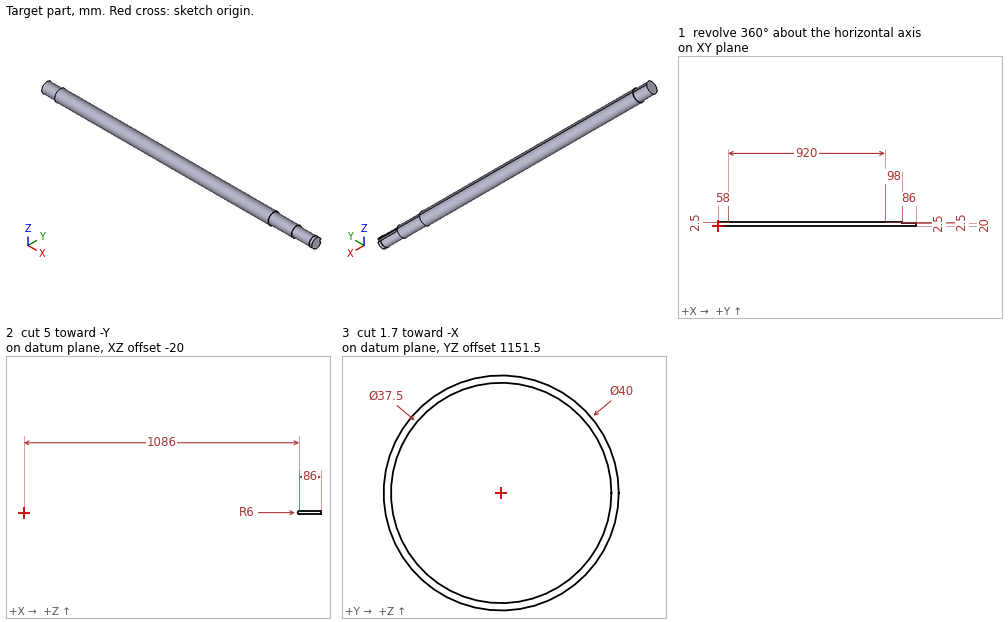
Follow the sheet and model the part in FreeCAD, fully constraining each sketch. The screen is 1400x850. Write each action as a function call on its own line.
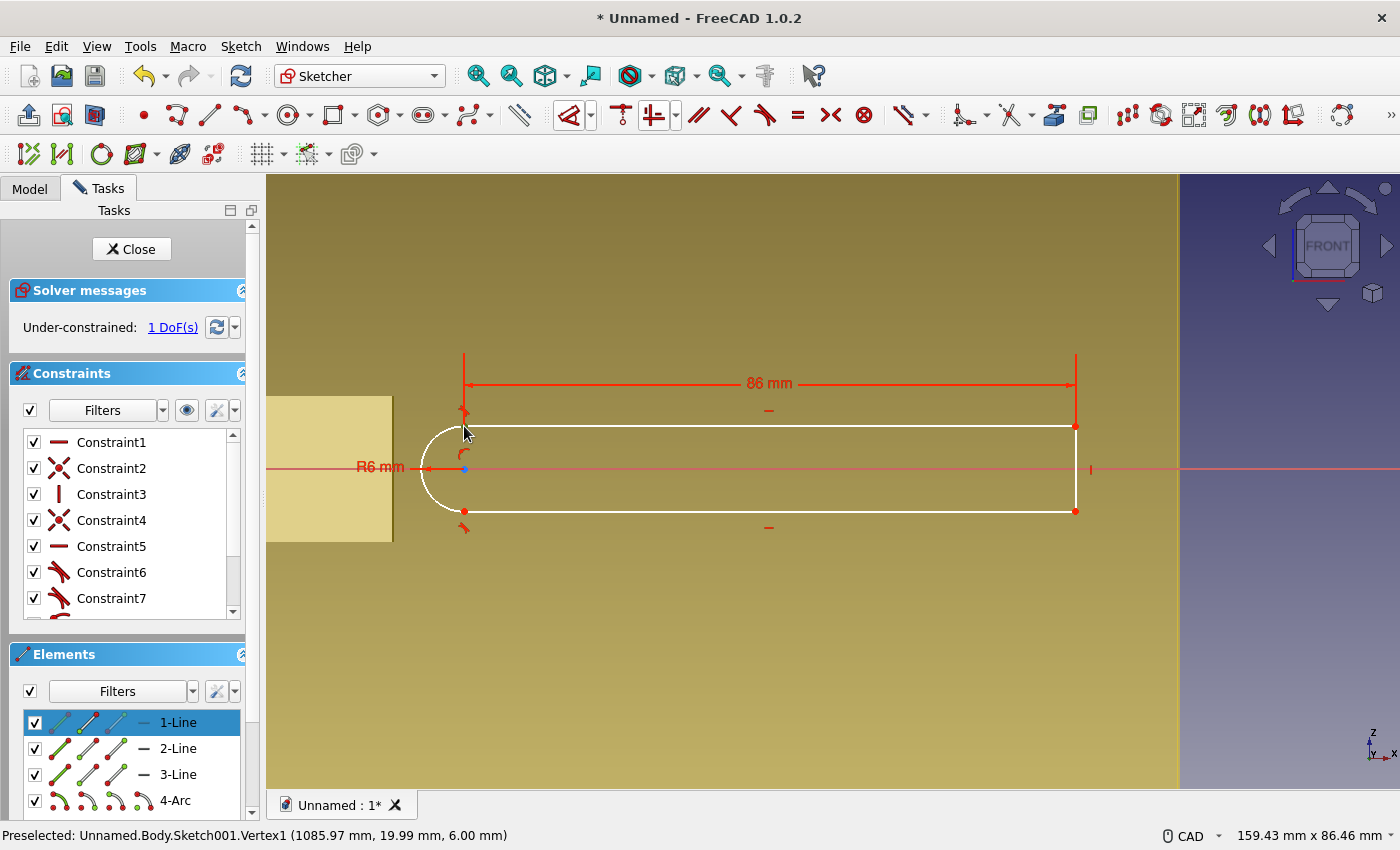
click(590, 116)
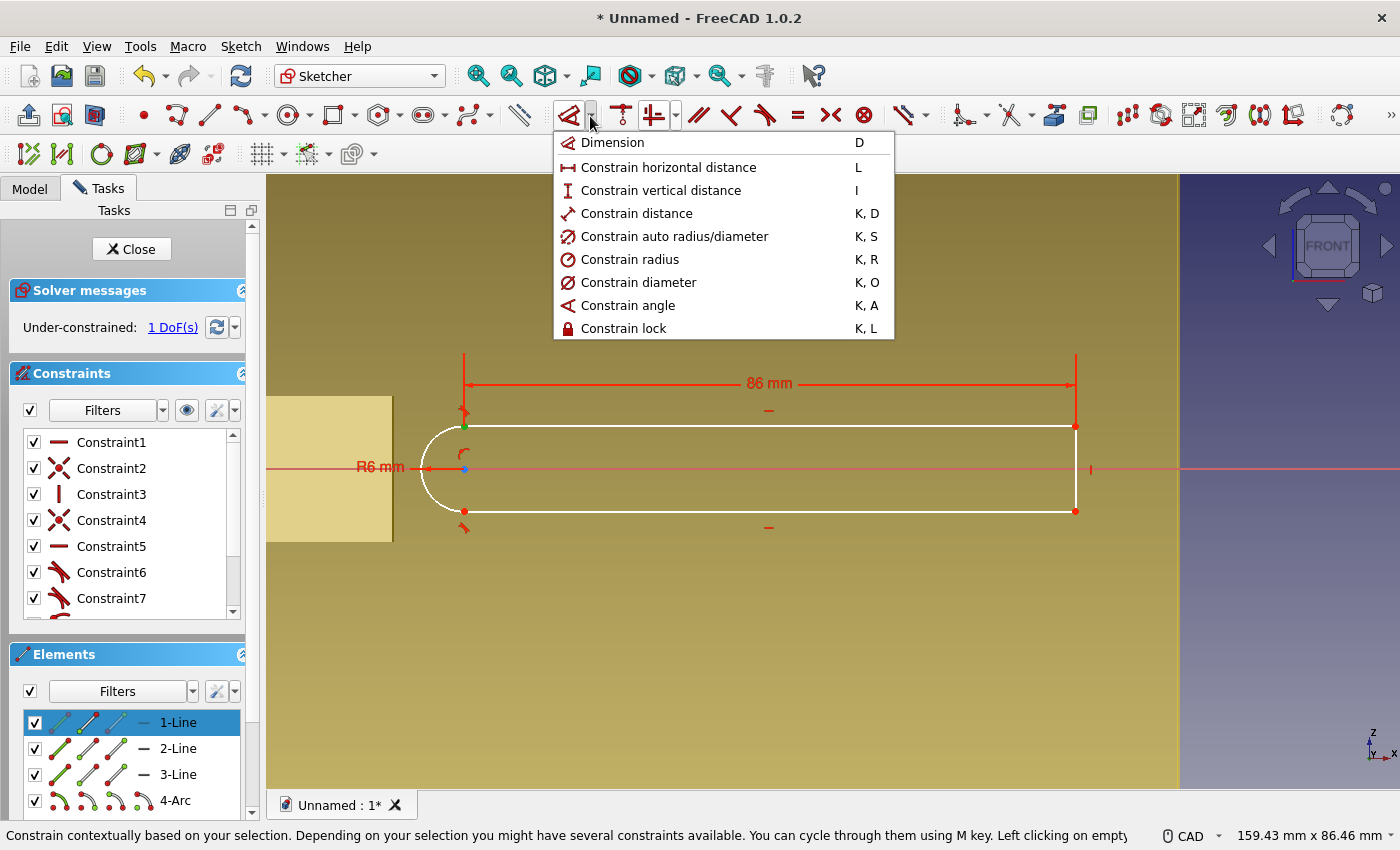
click(724, 168)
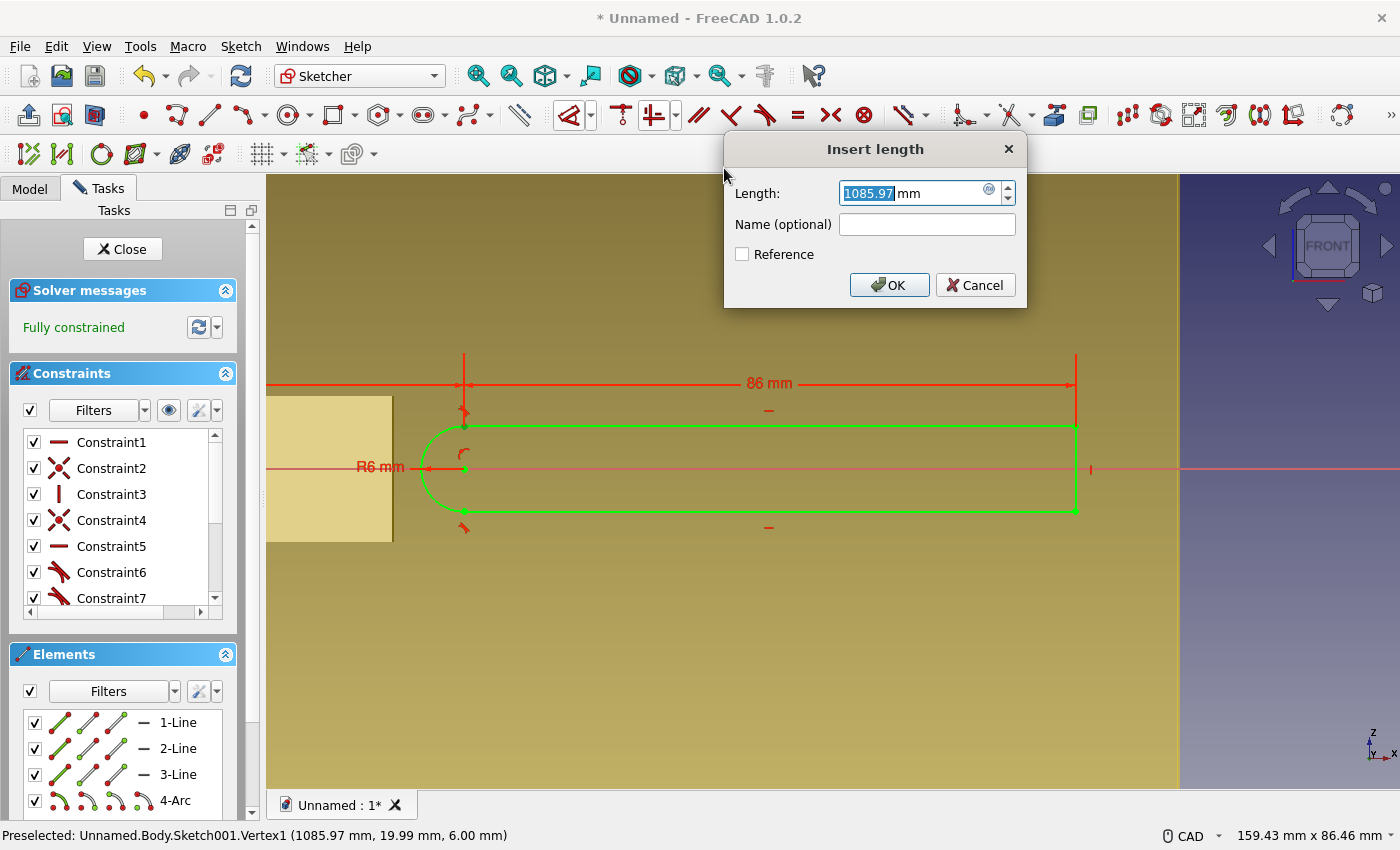
text(1086)
key(Return)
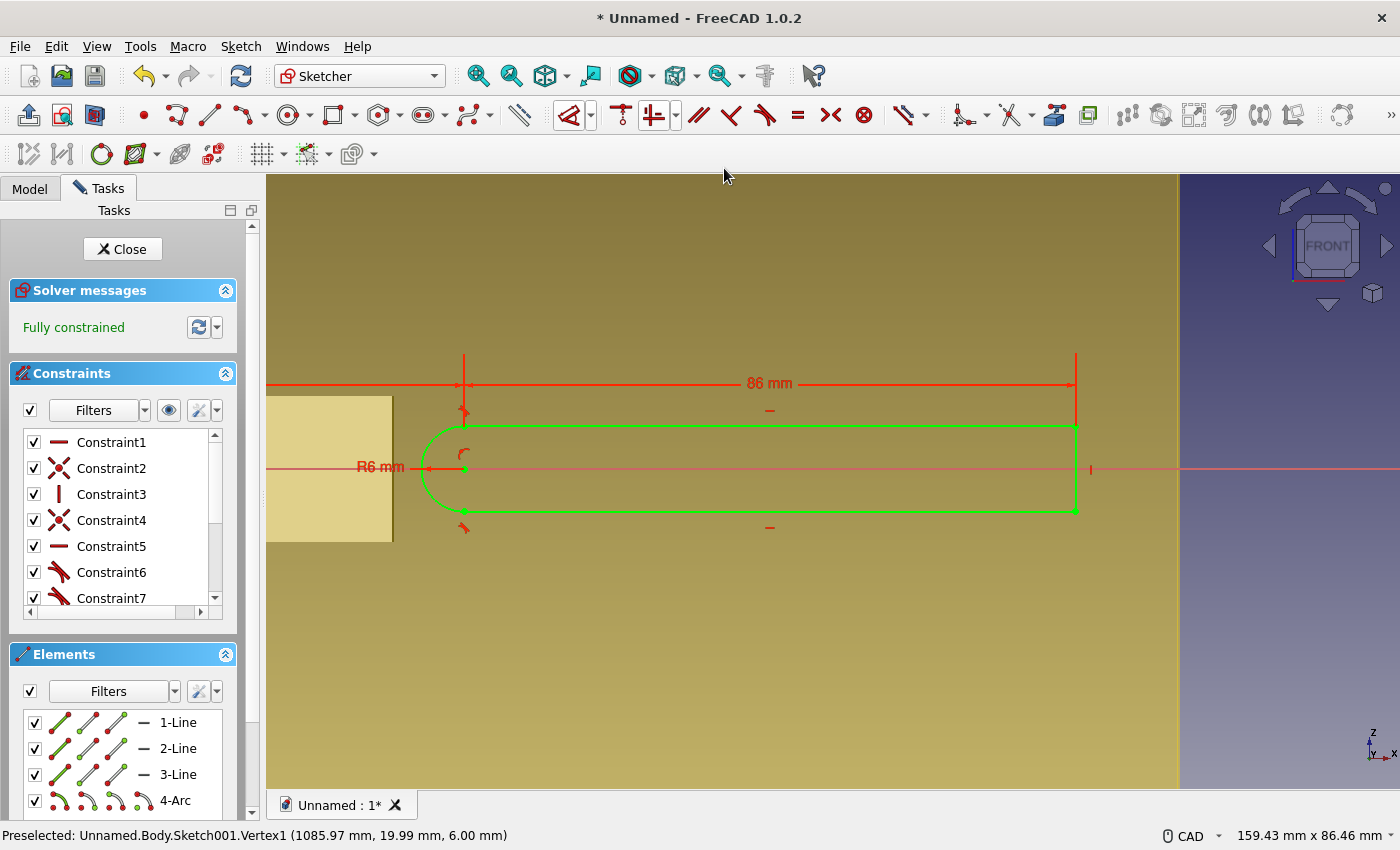
click(123, 249)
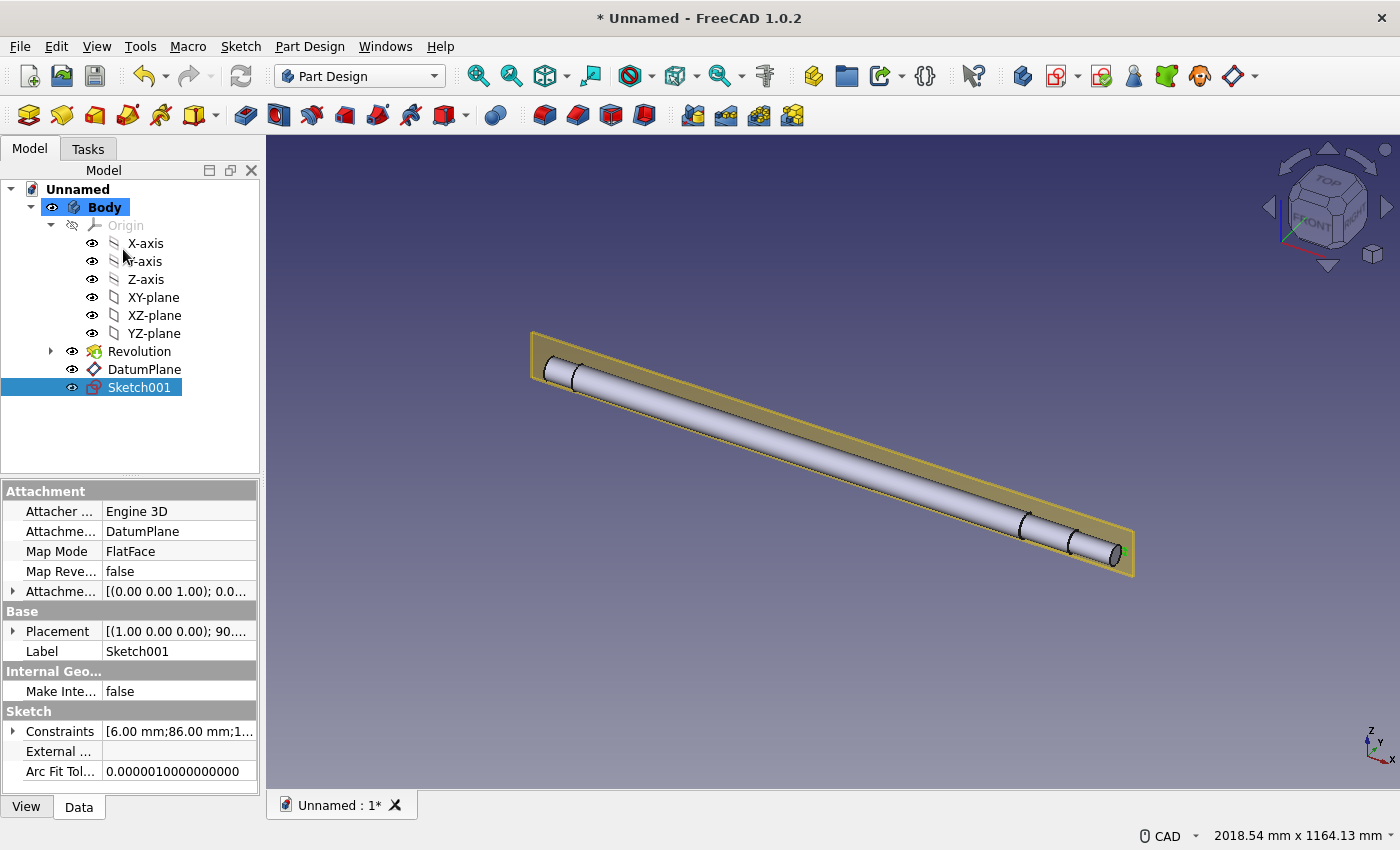
click(246, 116)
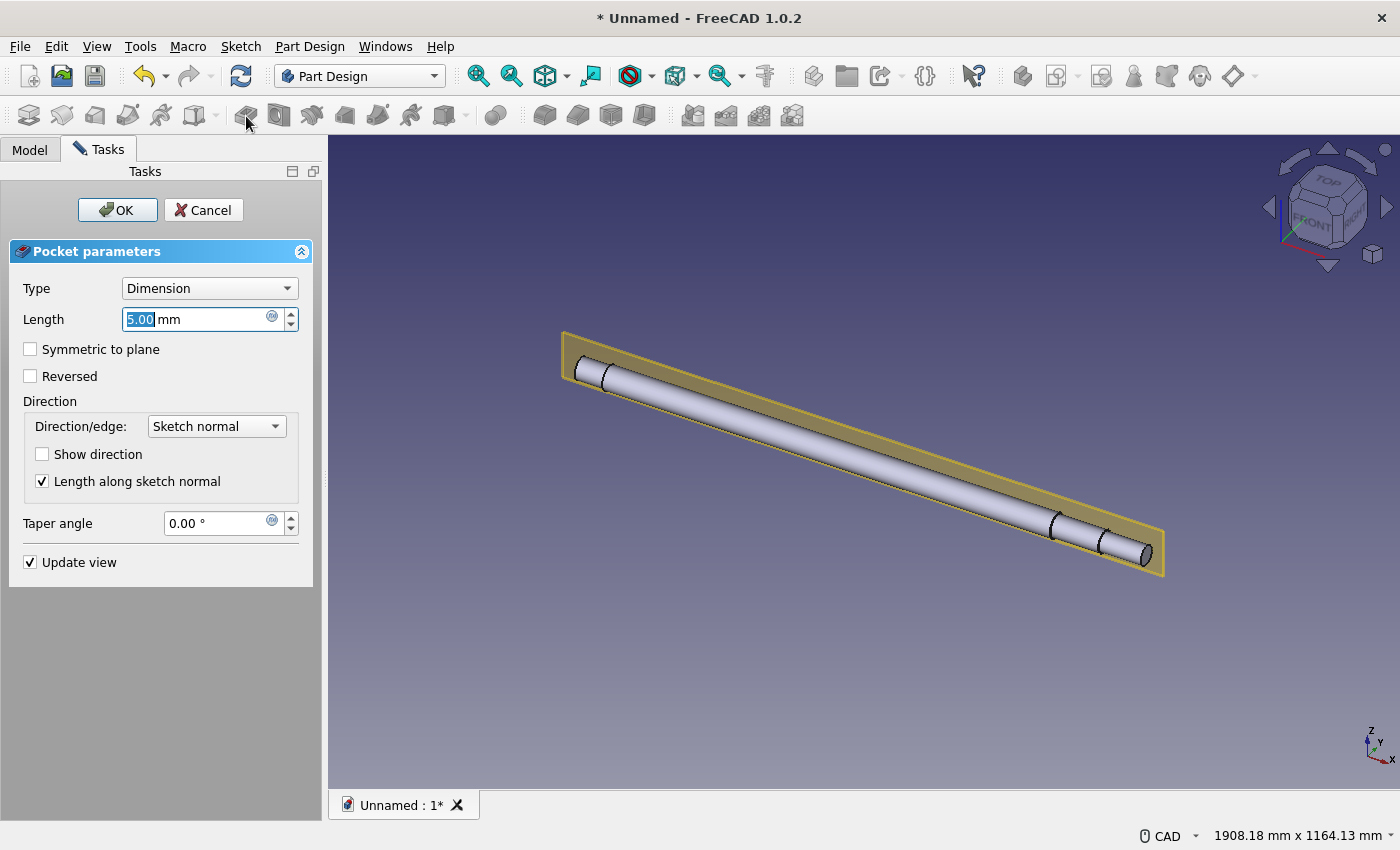
text(5)
key(Tab)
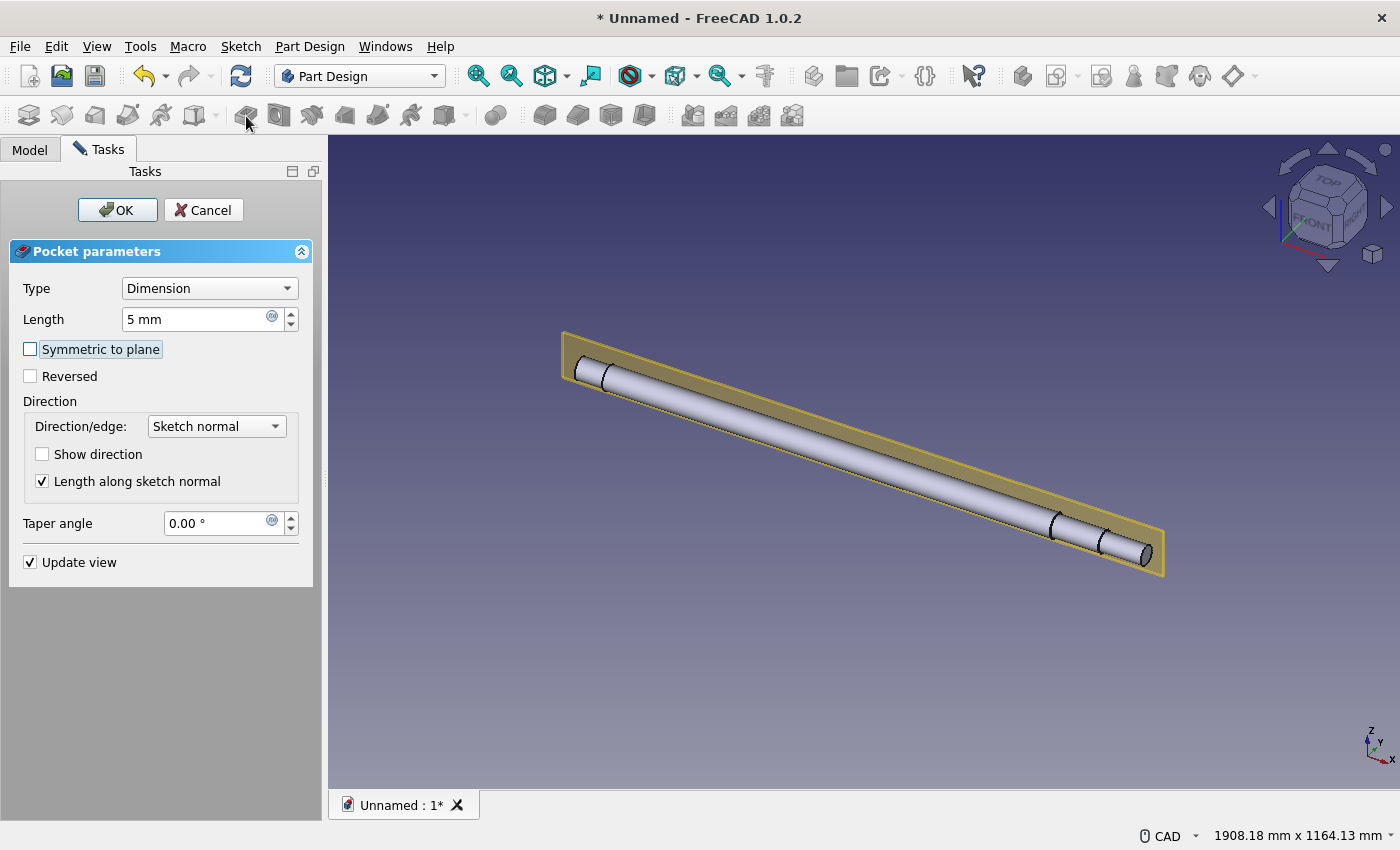
click(31, 376)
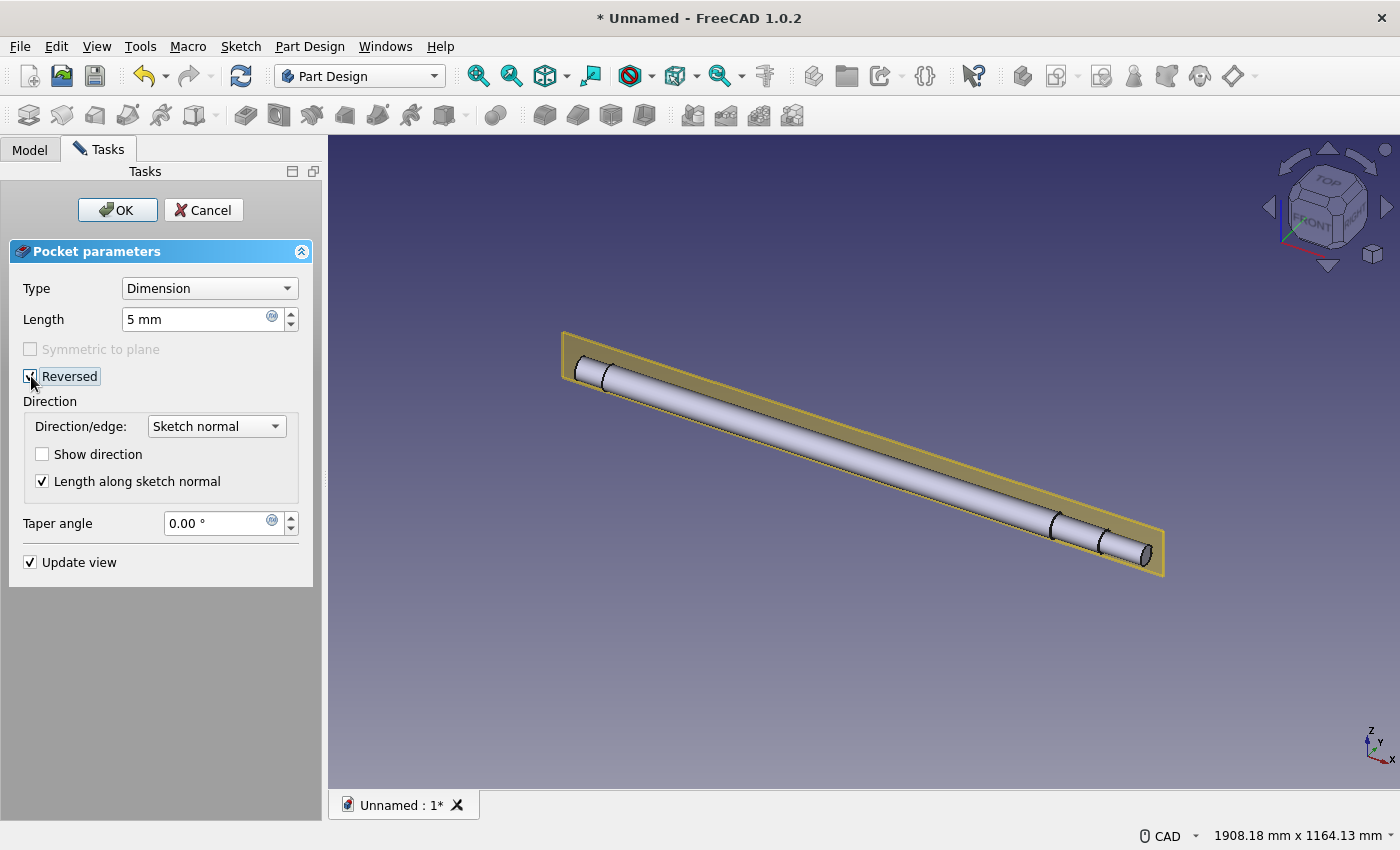
click(118, 210)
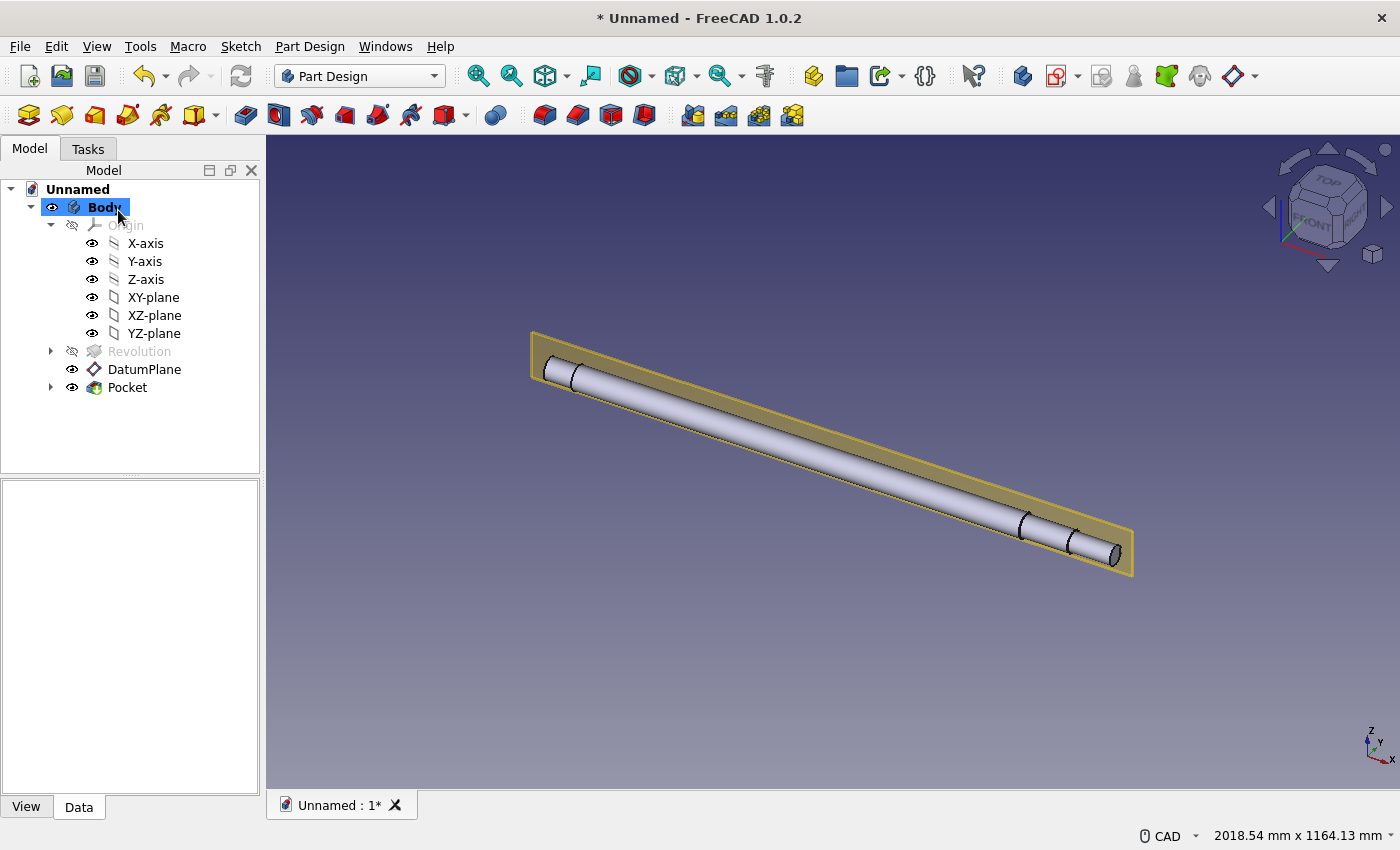
click(117, 369)
key(space)